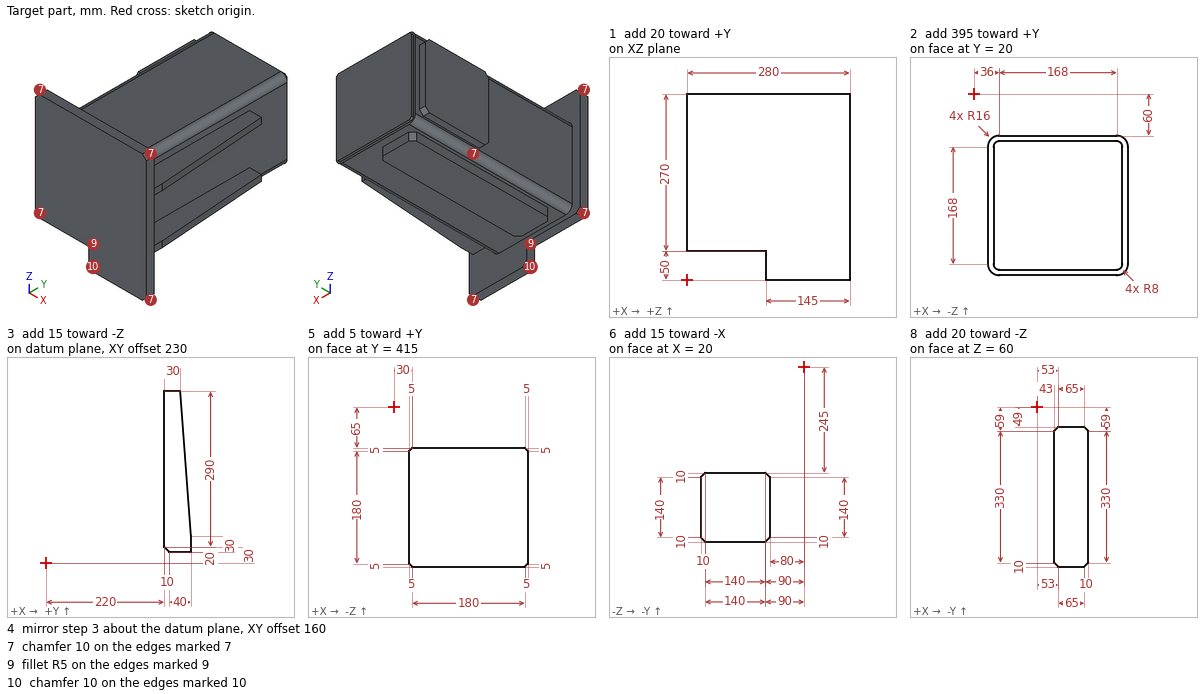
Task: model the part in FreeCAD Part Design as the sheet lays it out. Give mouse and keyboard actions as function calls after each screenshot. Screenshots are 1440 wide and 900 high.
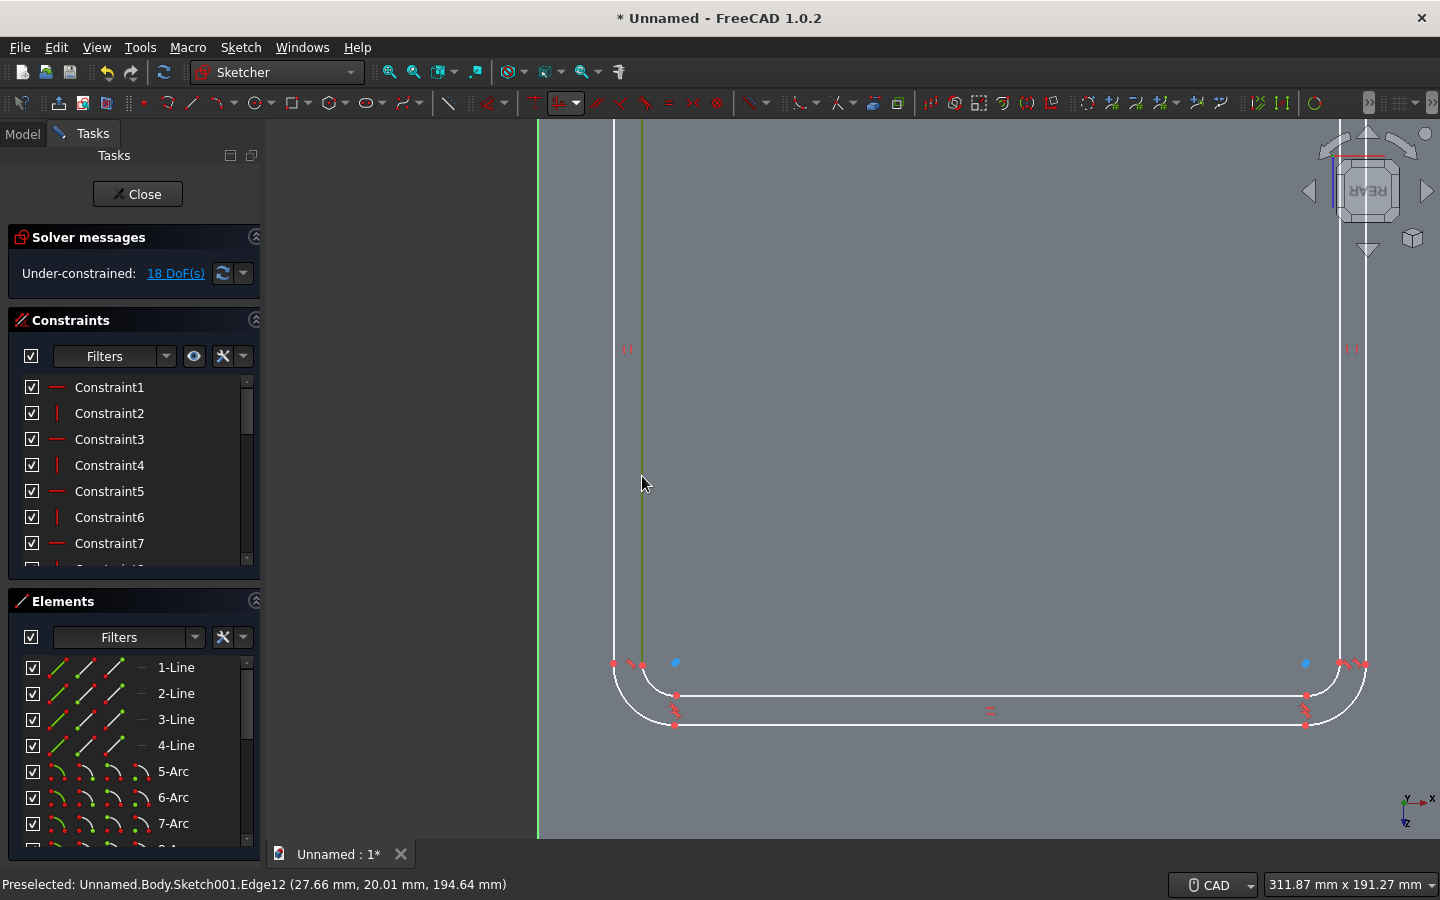
click(647, 680)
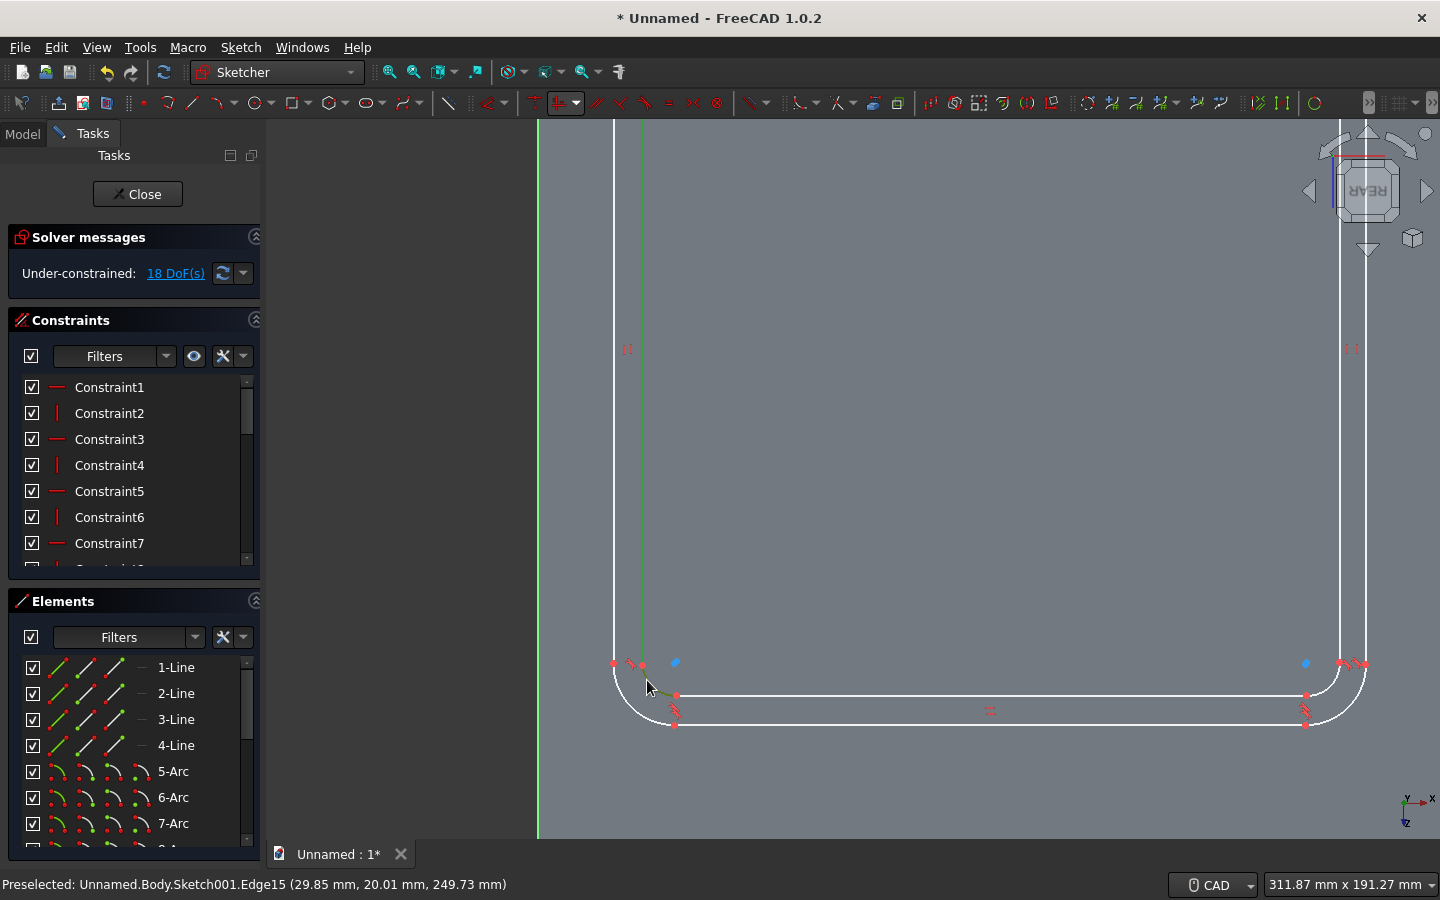
click(646, 104)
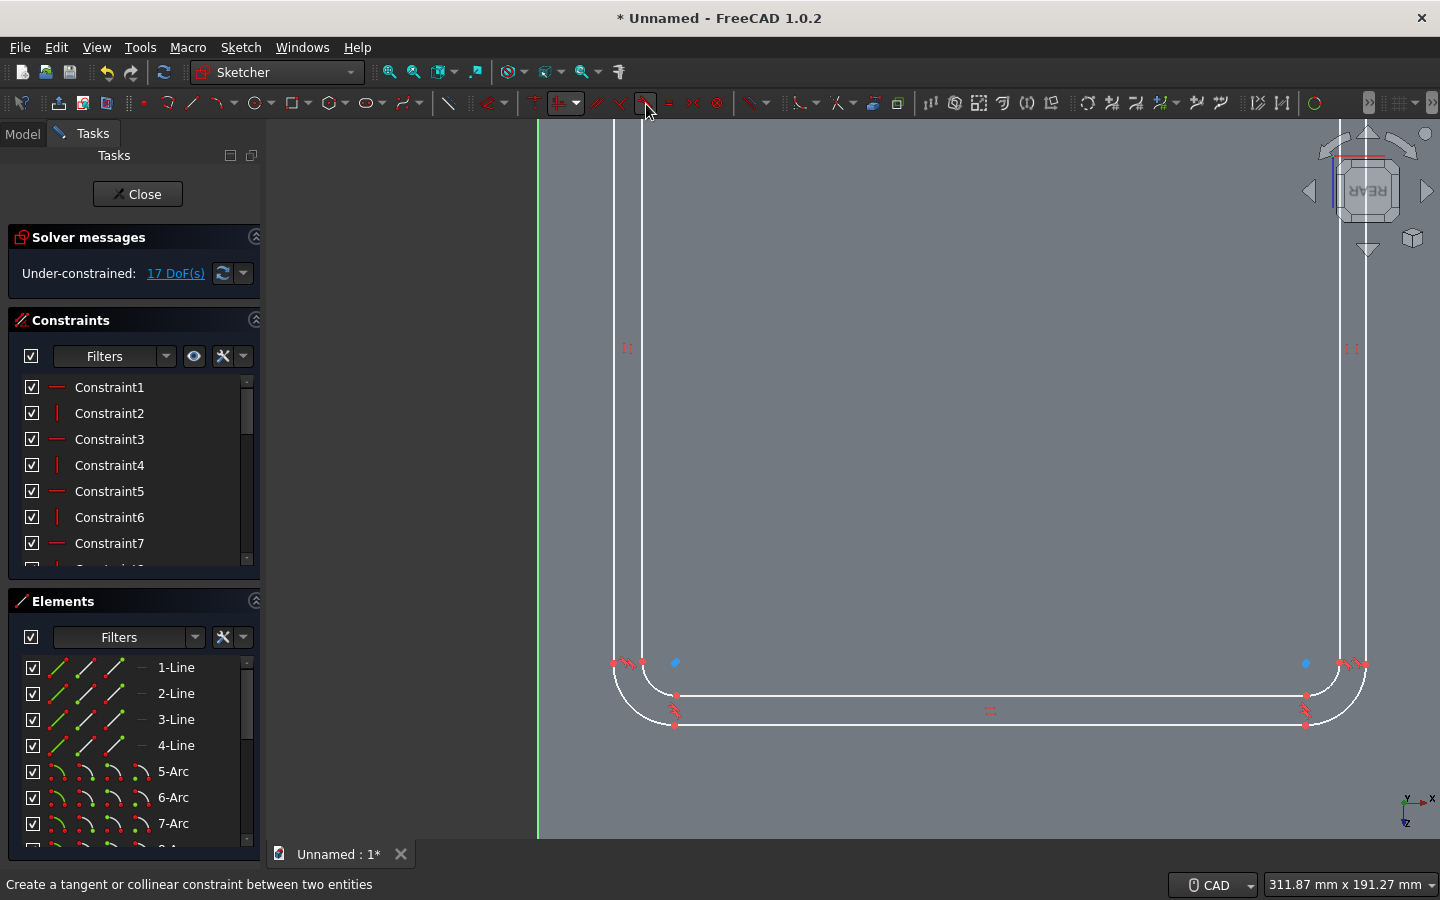
click(642, 473)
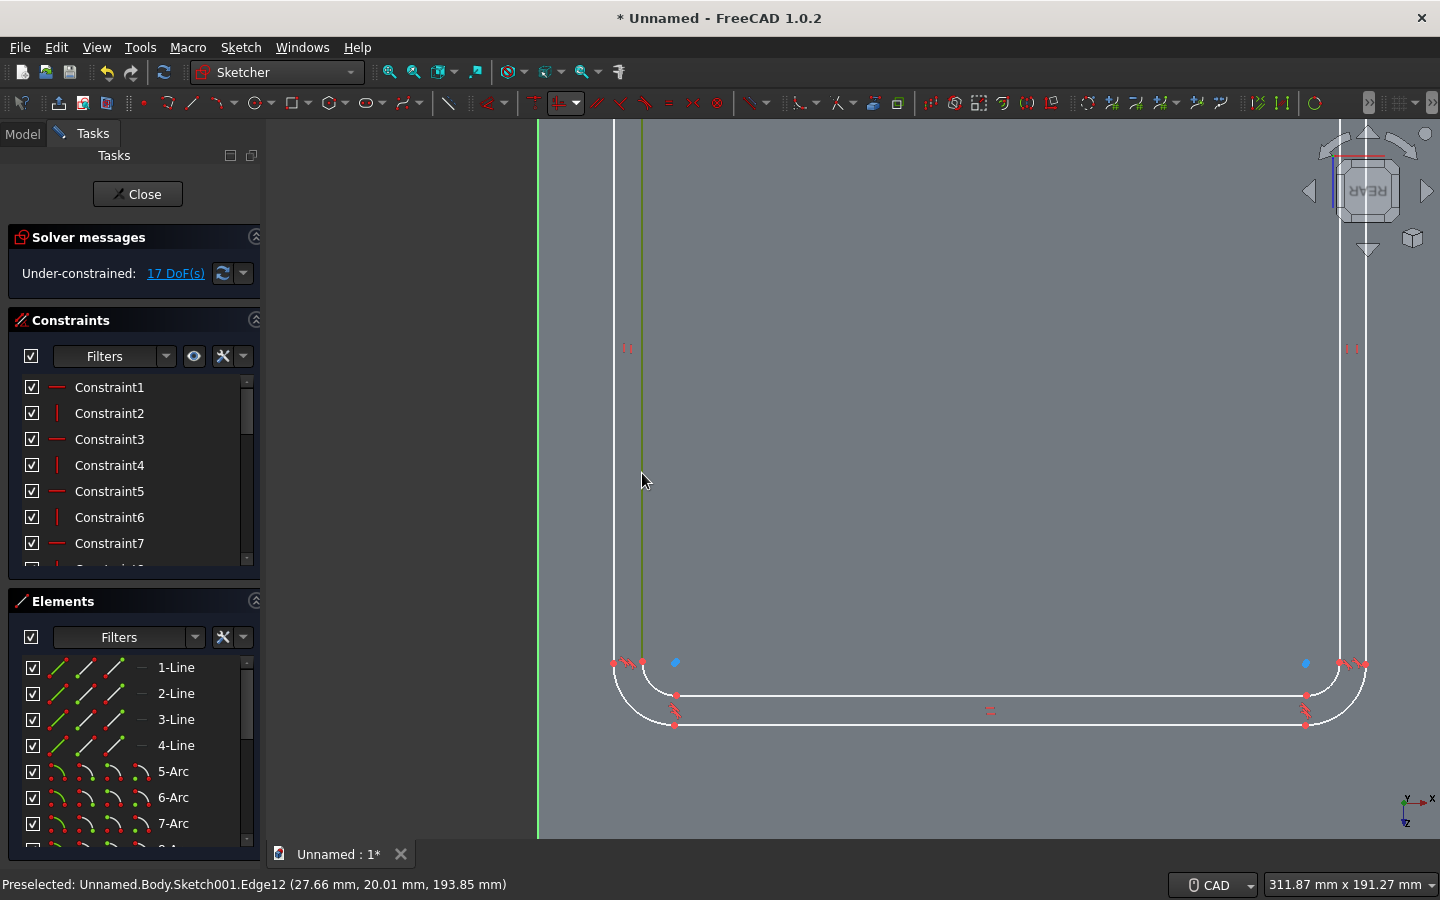
scroll(648, 679, down, 4)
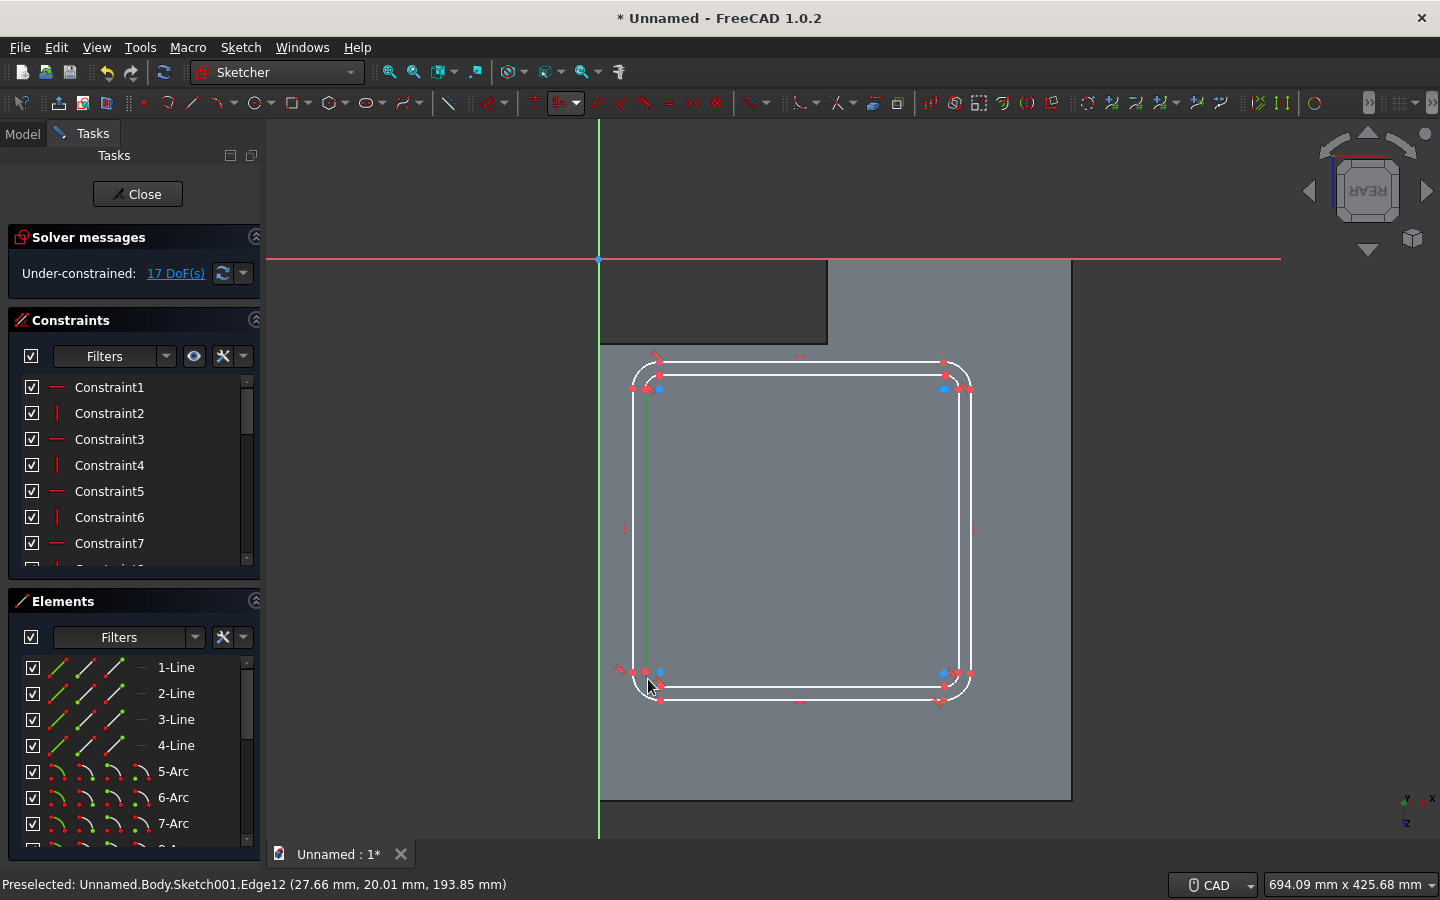
scroll(653, 377, up, 4)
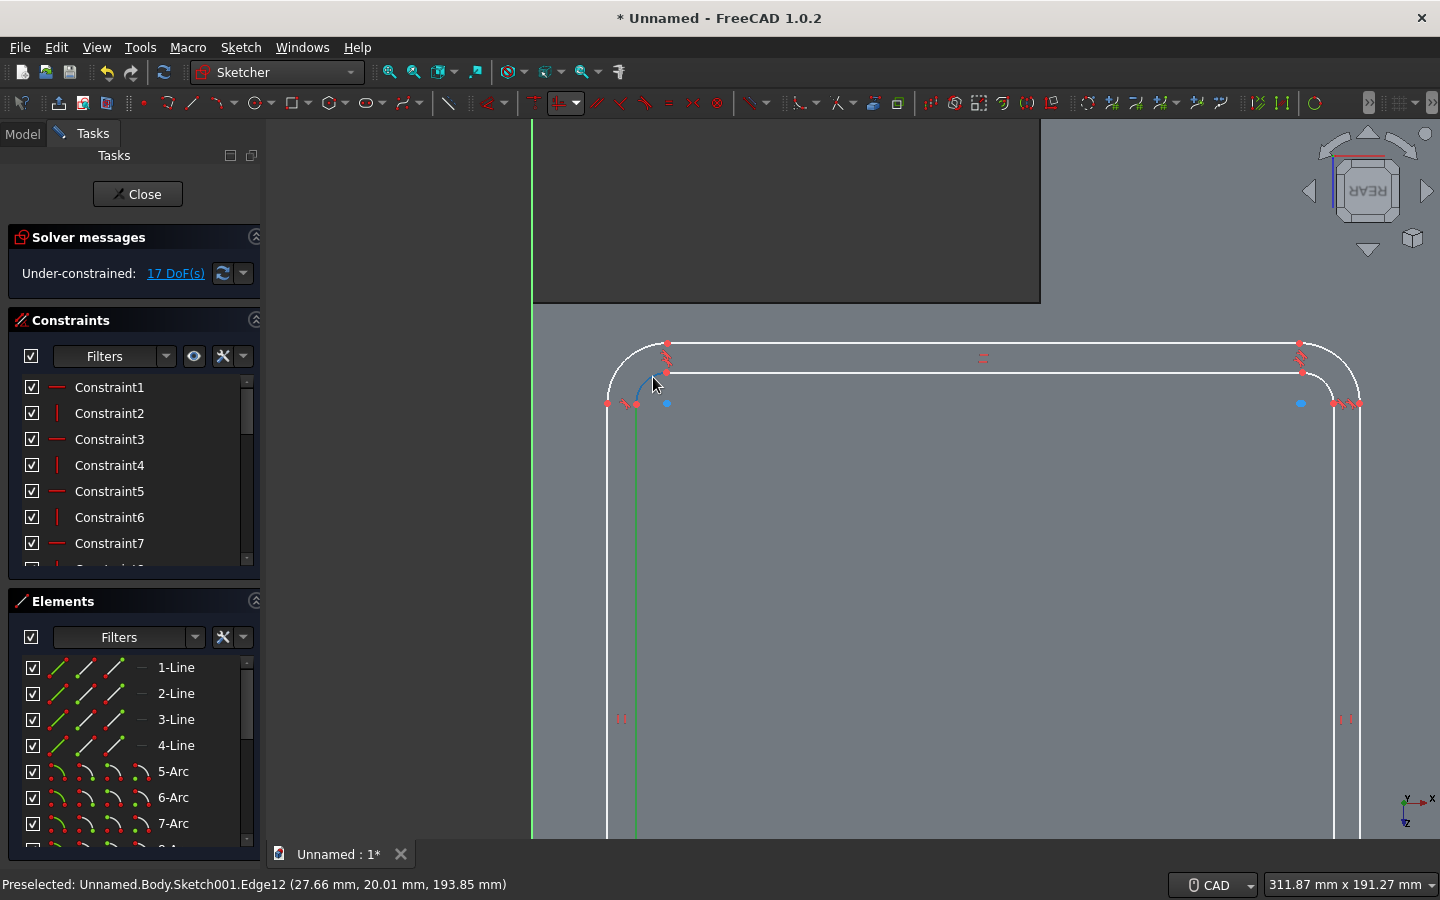
click(653, 376)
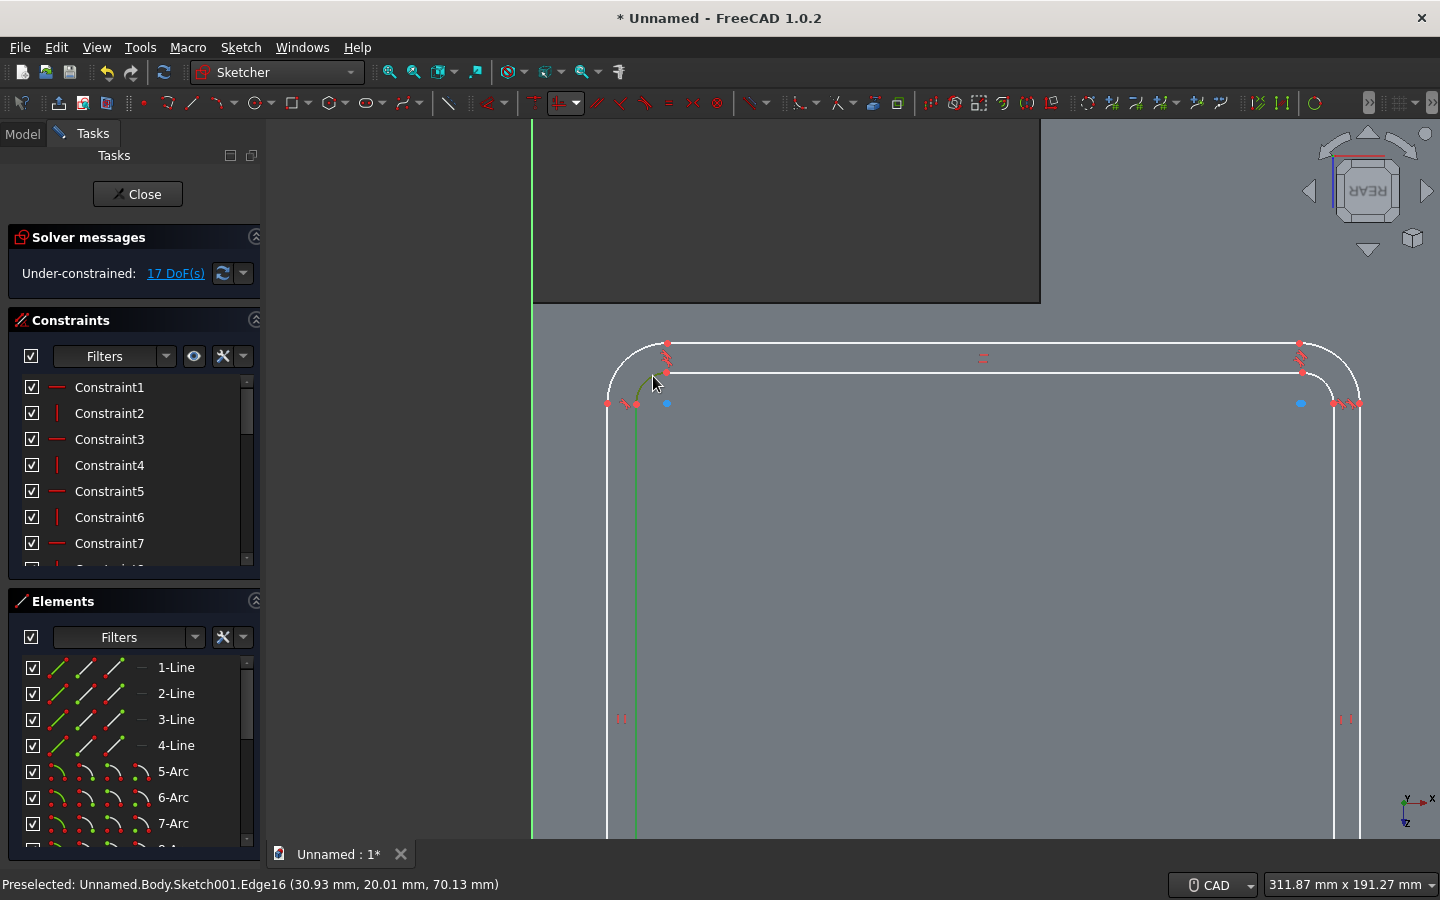
key(t)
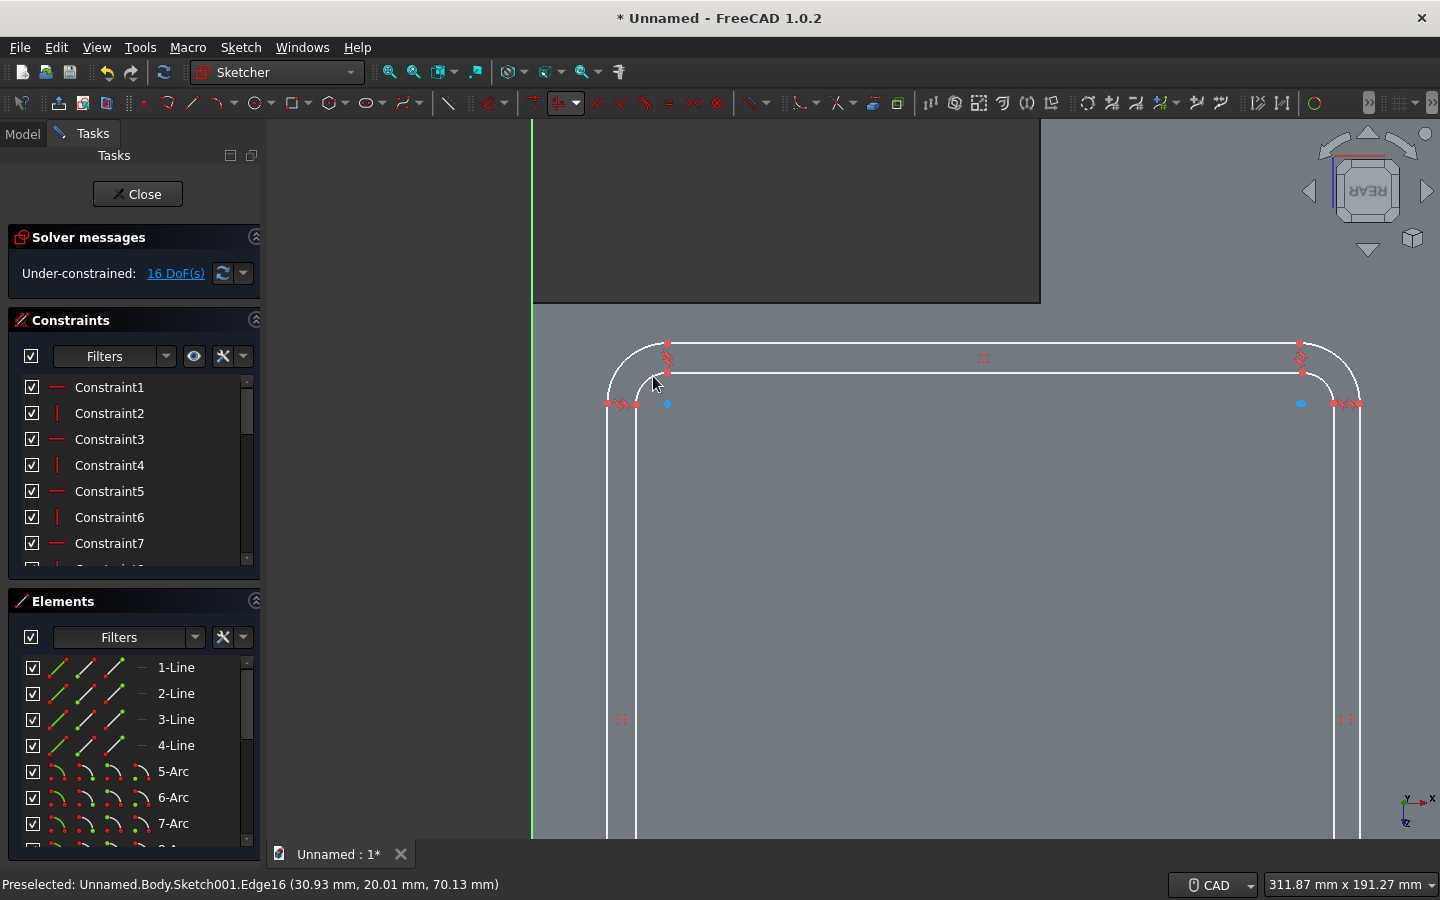
scroll(653, 377, down, 4)